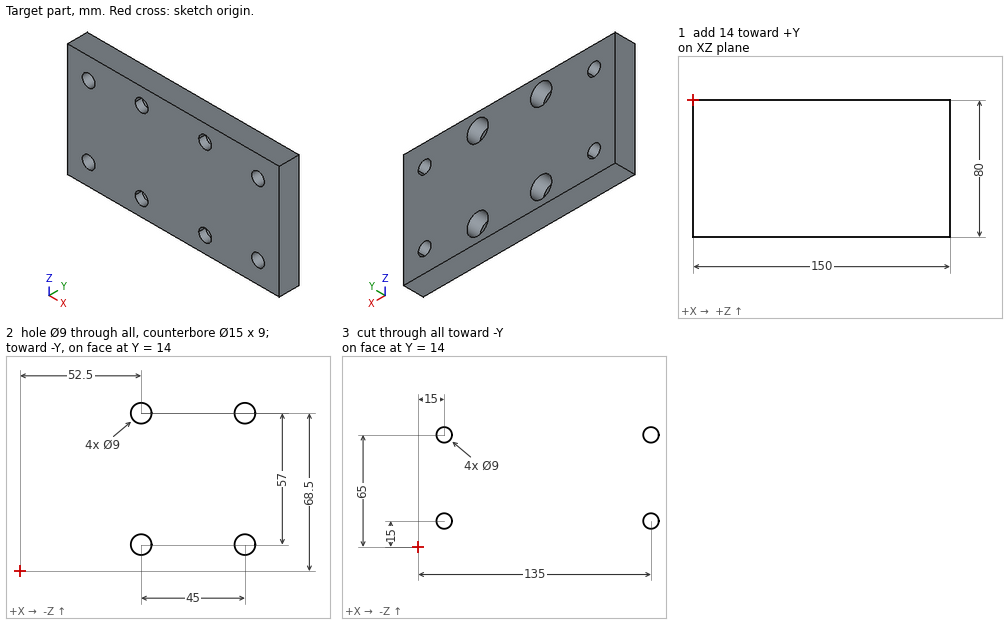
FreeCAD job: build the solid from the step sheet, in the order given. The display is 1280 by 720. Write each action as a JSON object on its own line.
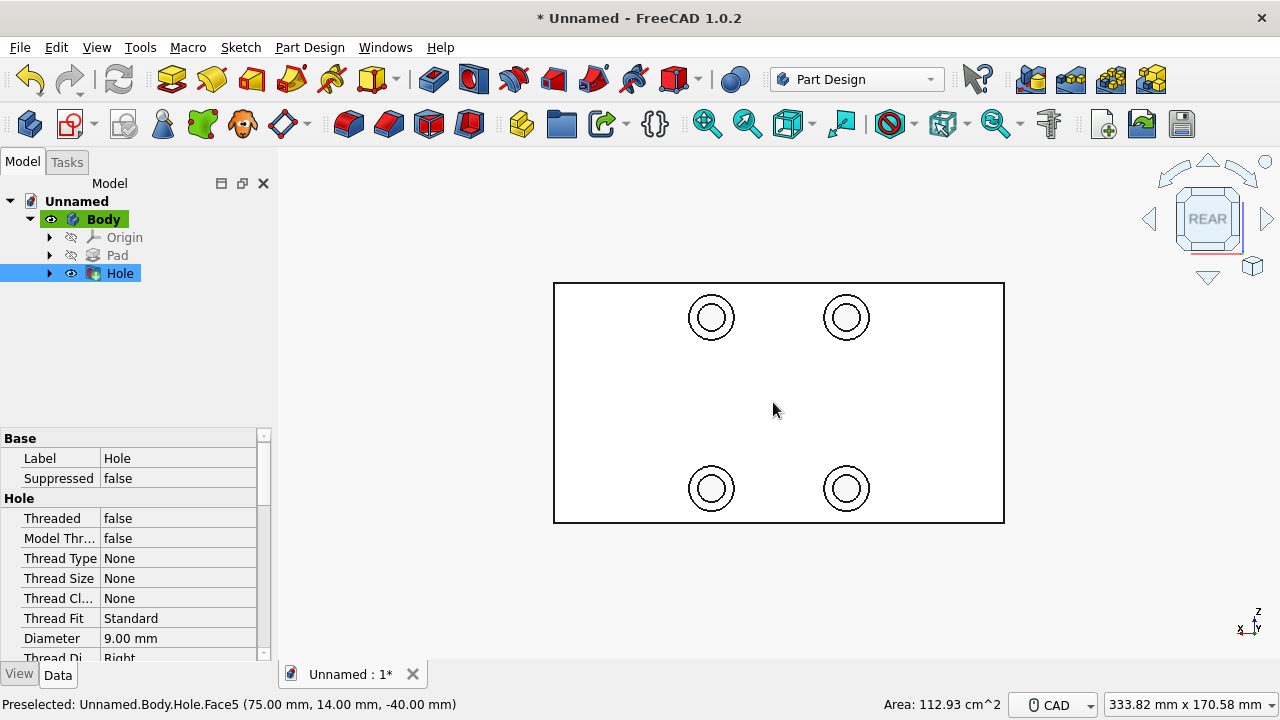
{"action": "left_click", "coordinate": [70, 124]}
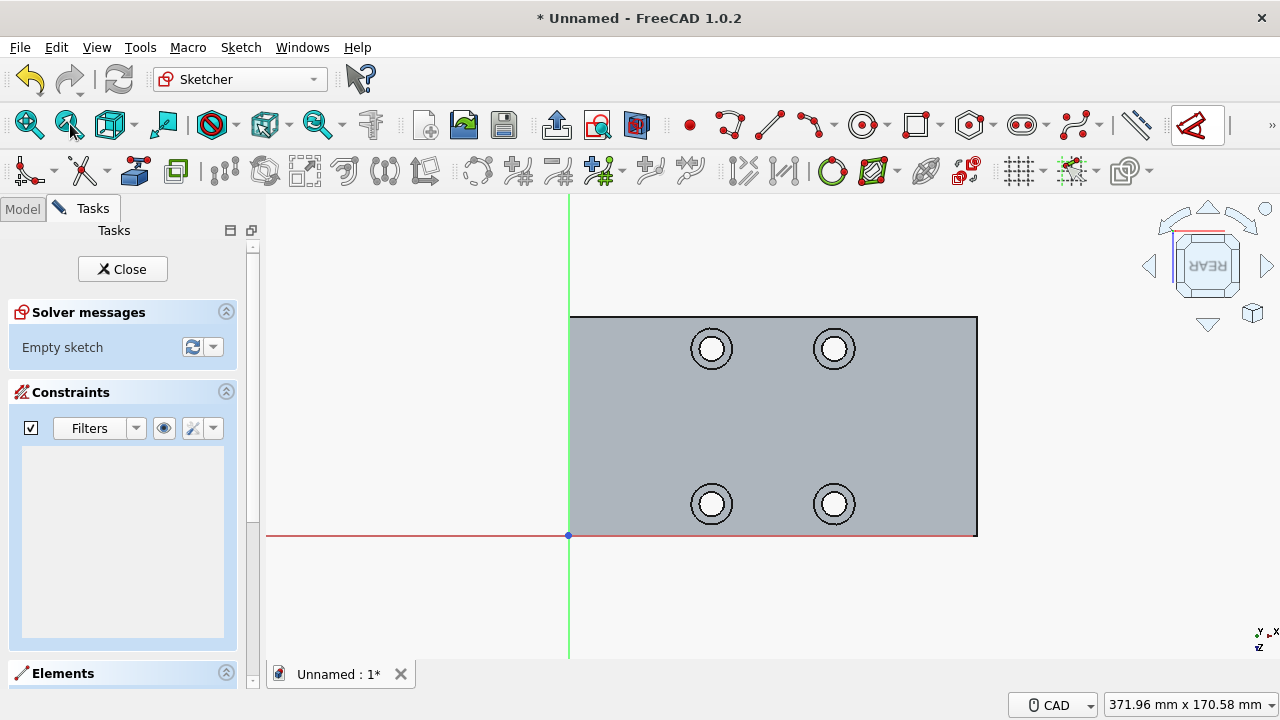
{"action": "scroll", "coordinate": [869, 470], "scroll_direction": "up", "scroll_amount": 2}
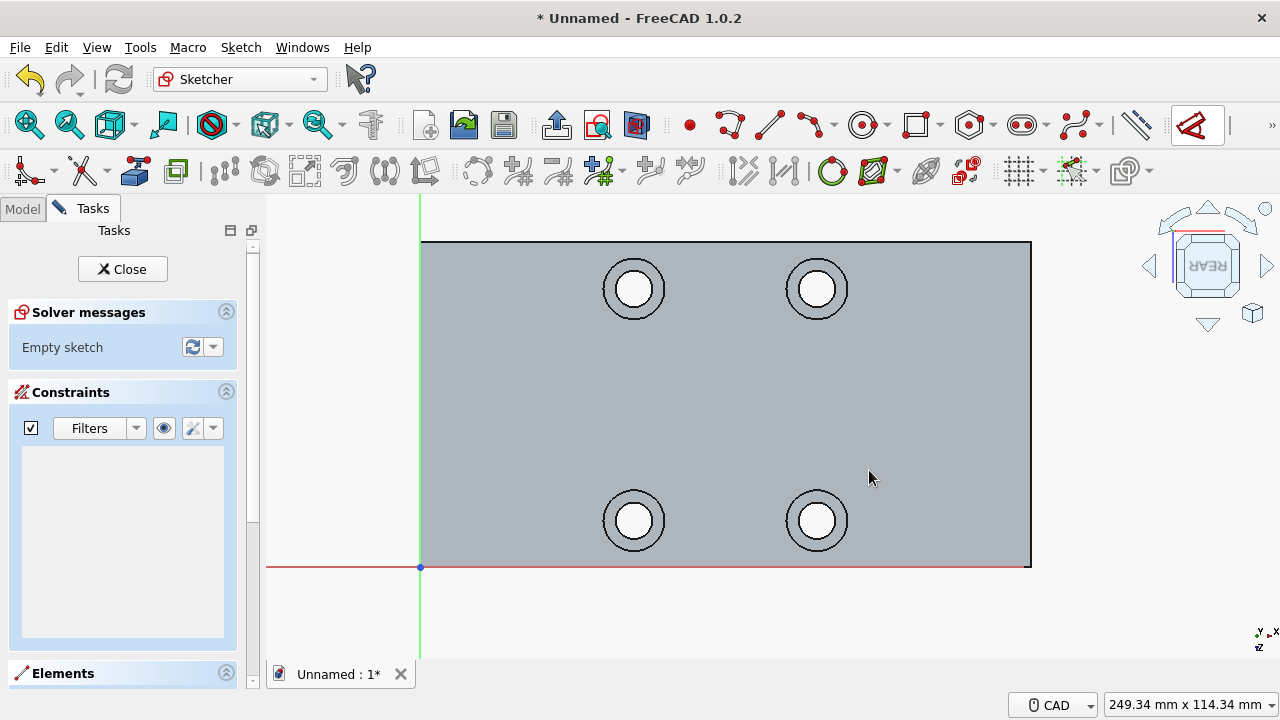
{"action": "left_click", "coordinate": [864, 126]}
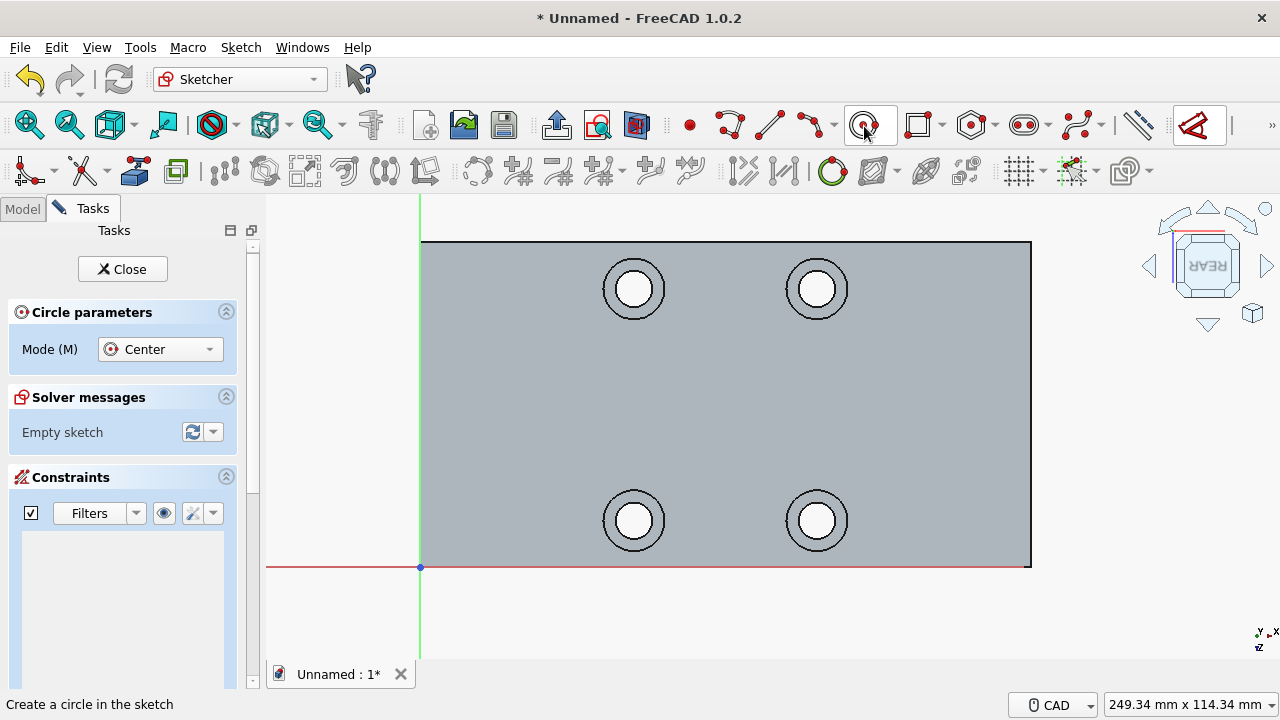
{"action": "scroll", "coordinate": [481, 303], "scroll_direction": "up", "scroll_amount": 2}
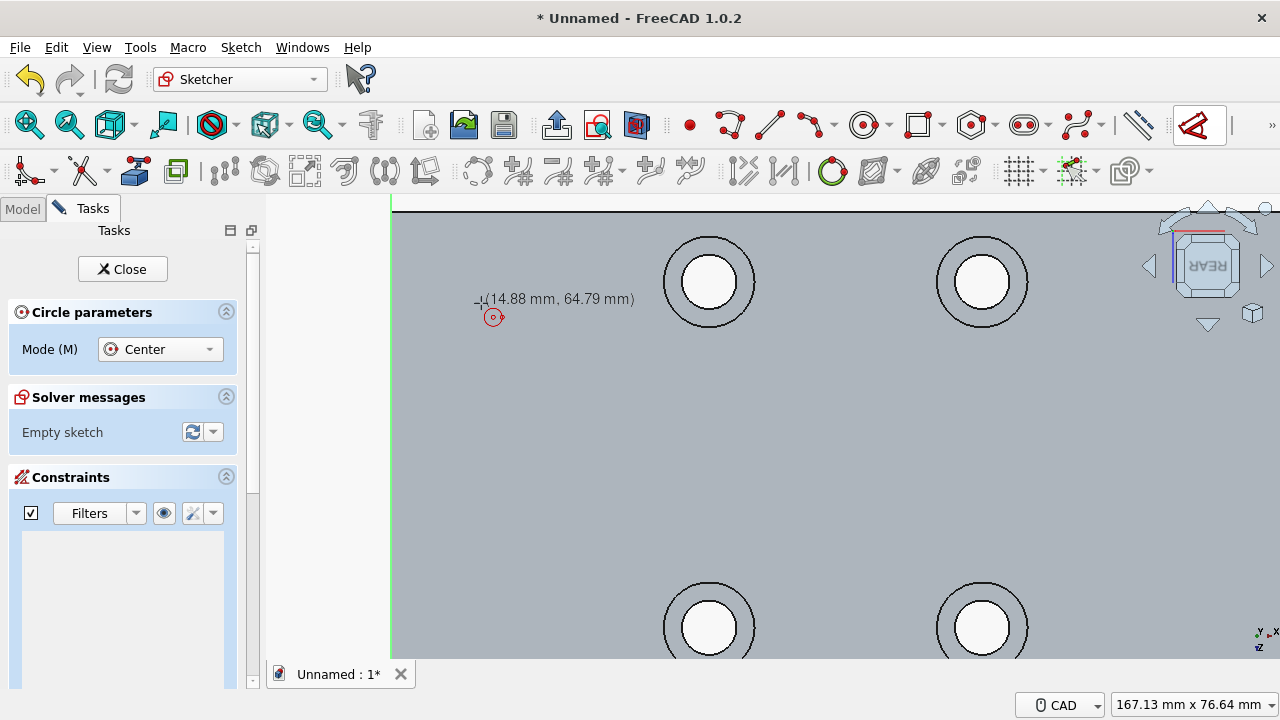
{"action": "left_click", "coordinate": [482, 303]}
{"action": "mouse_move", "coordinate": [501, 284]}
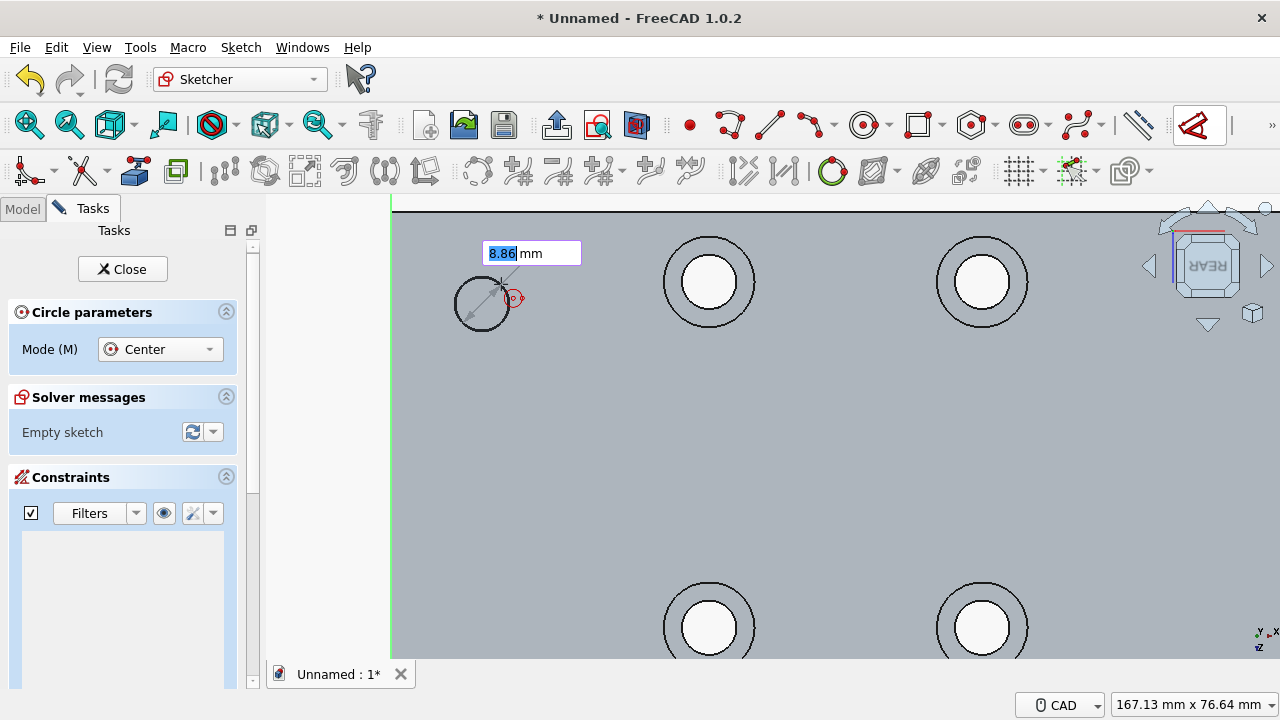
{"action": "type", "text": "9"}
{"action": "key", "text": "Return"}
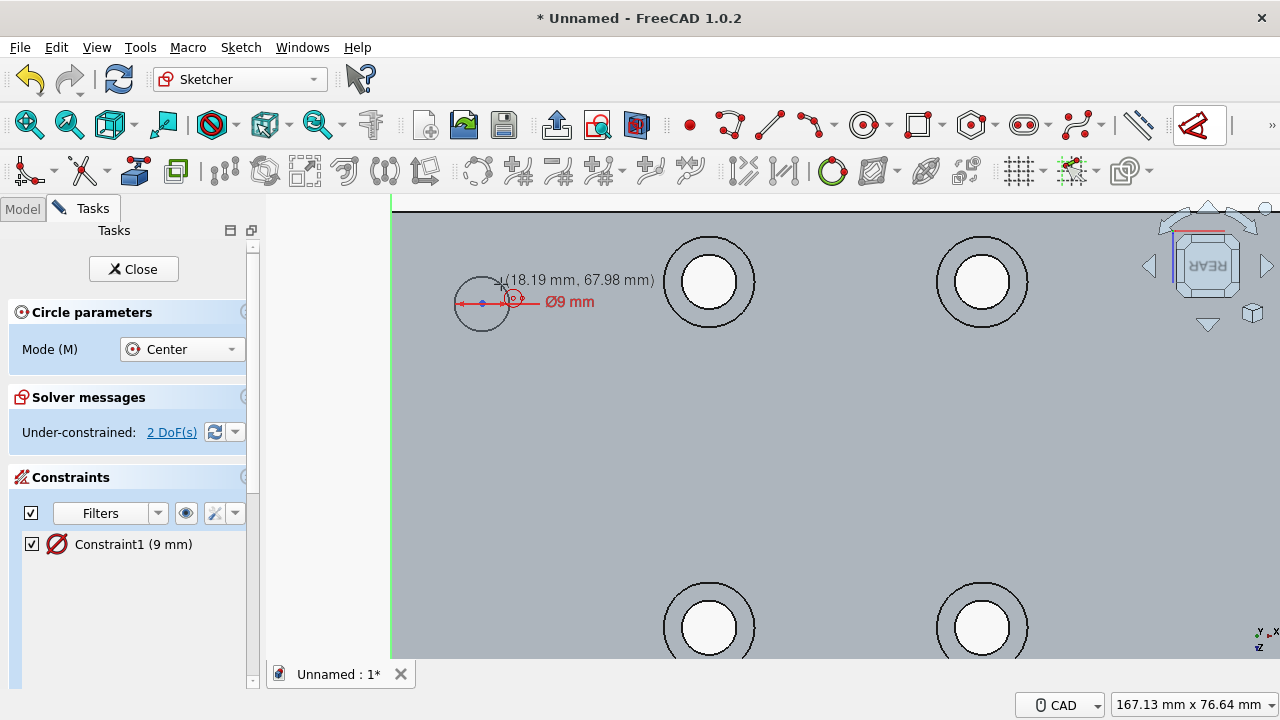
{"action": "left_click", "coordinate": [482, 606]}
{"action": "mouse_move", "coordinate": [501, 587]}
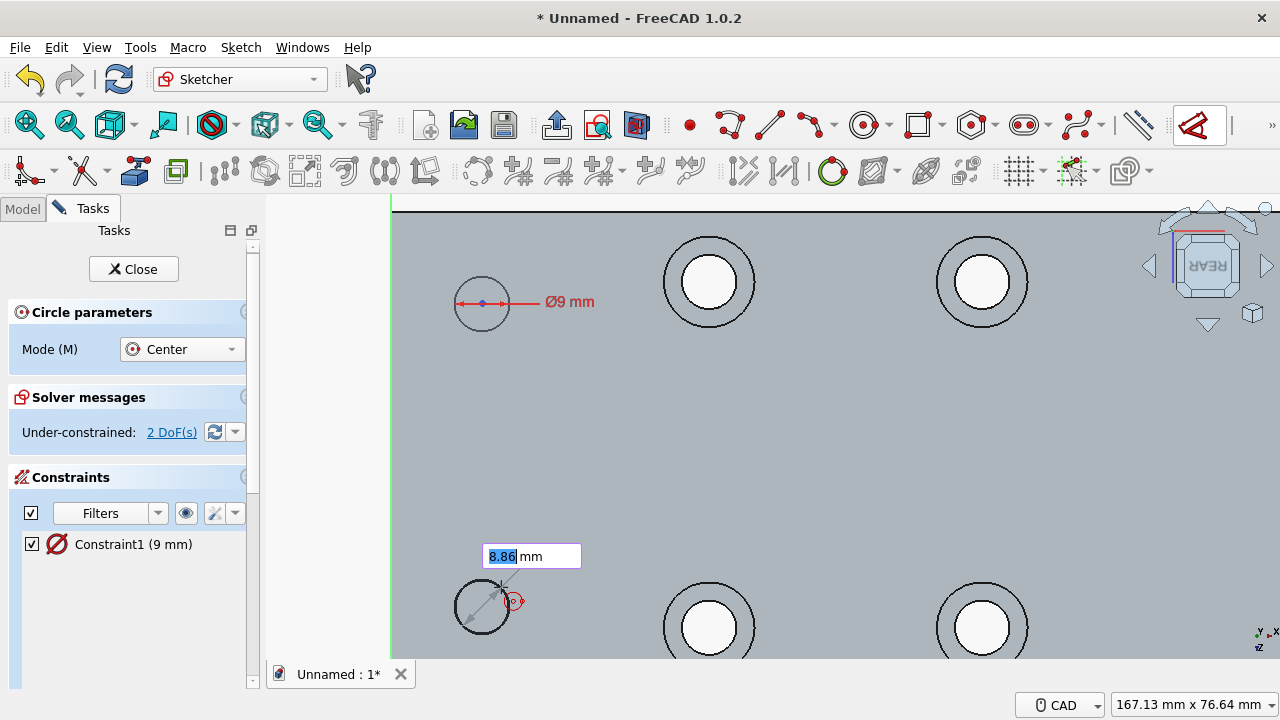
{"action": "type", "text": "9"}
{"action": "key", "text": "Return"}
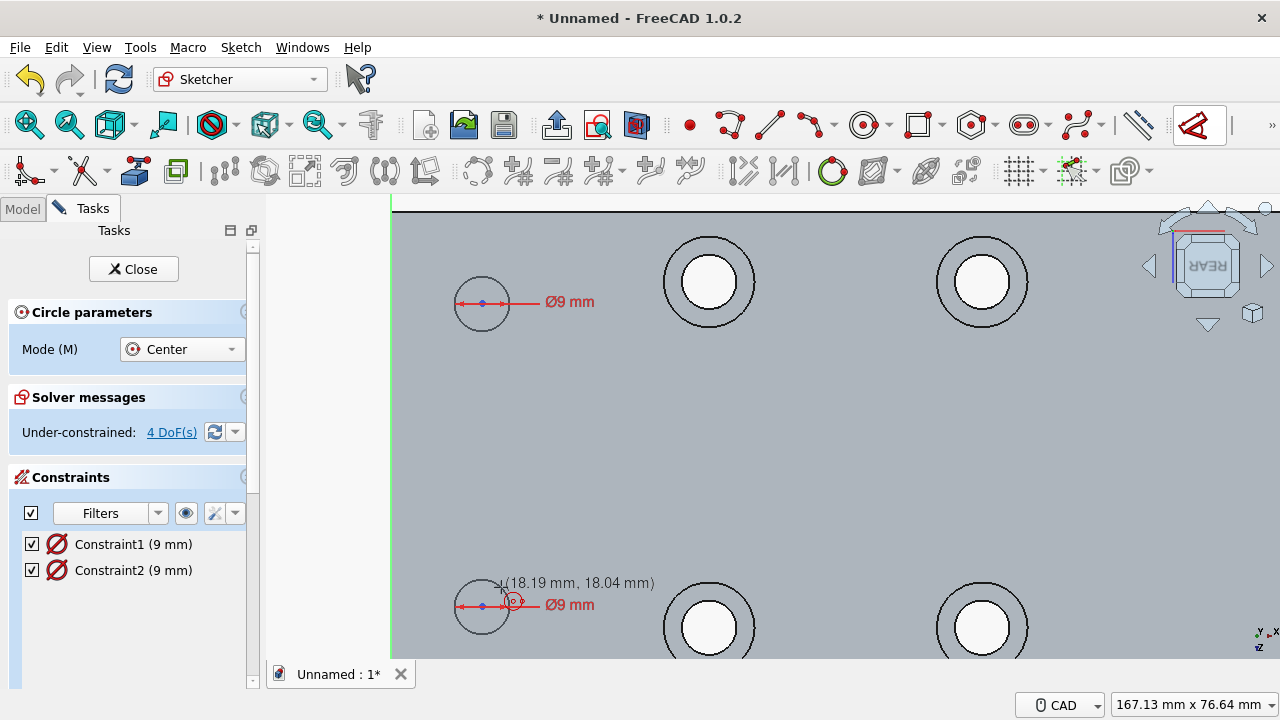
{"action": "scroll", "coordinate": [482, 304], "scroll_direction": "down", "scroll_amount": 2}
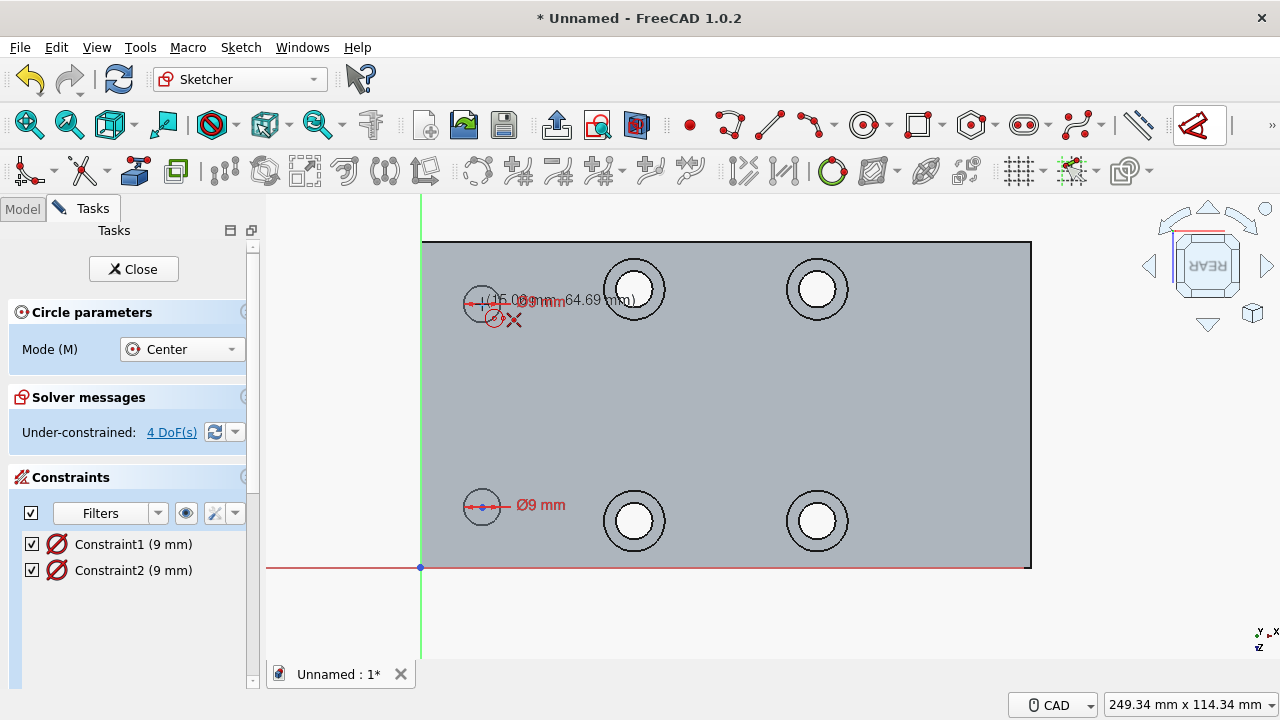
{"action": "scroll", "coordinate": [970, 507], "scroll_direction": "up", "scroll_amount": 2}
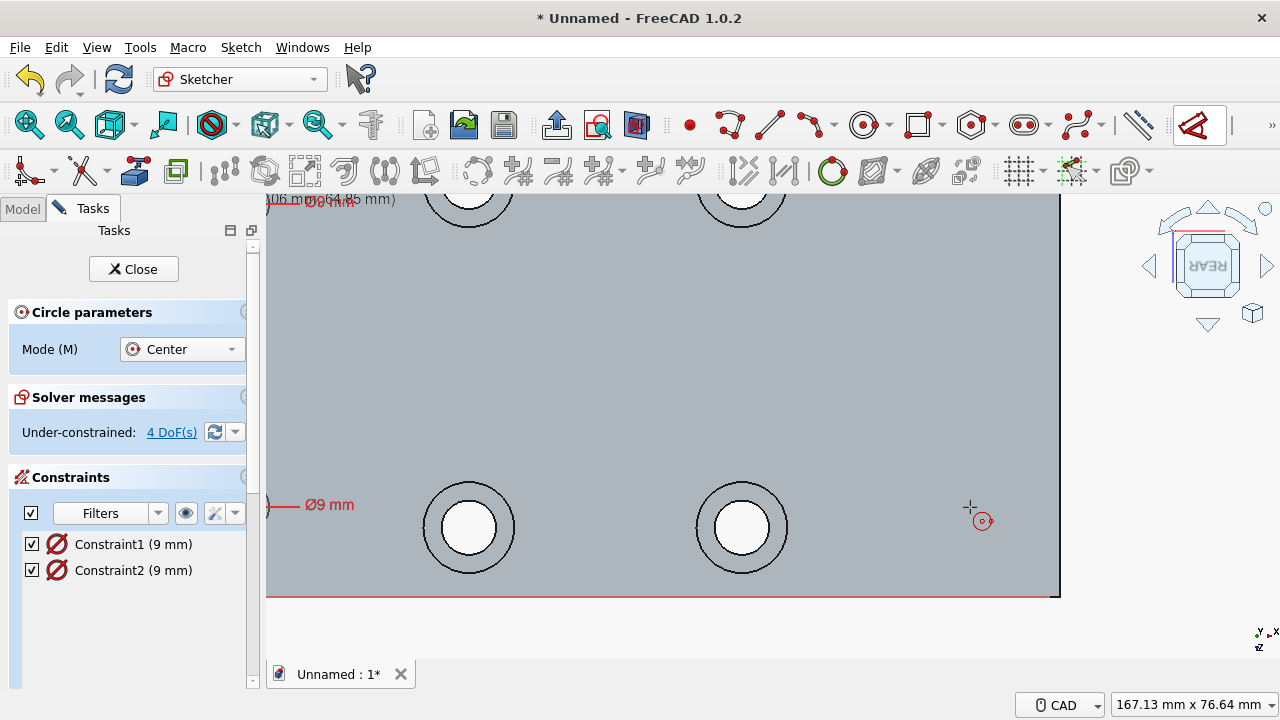
{"action": "left_click", "coordinate": [969, 506]}
{"action": "mouse_move", "coordinate": [989, 487]}